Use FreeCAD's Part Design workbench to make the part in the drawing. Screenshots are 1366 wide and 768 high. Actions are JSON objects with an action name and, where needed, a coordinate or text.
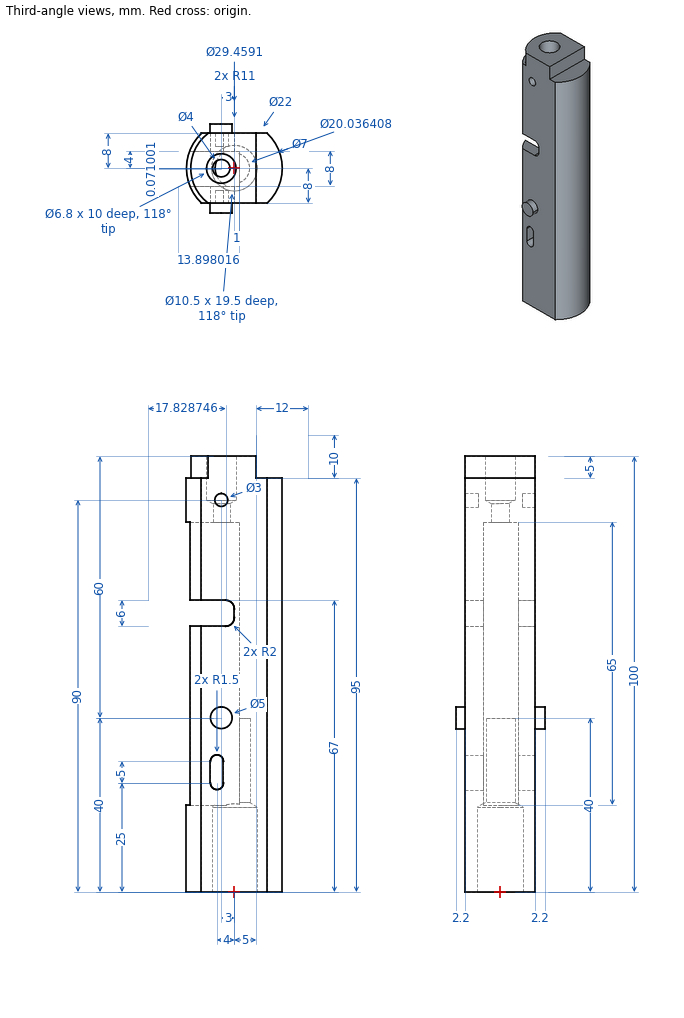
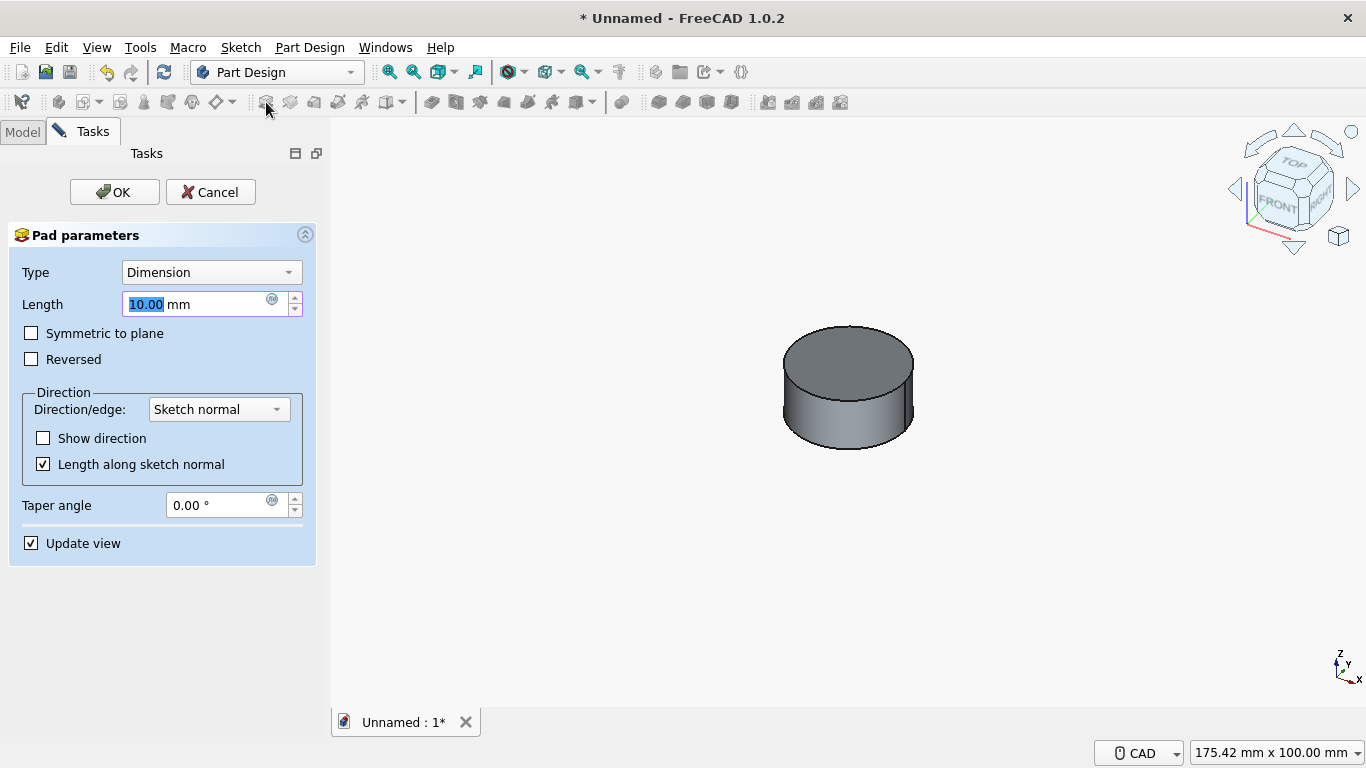
{"action": "type", "text": "100"}
{"action": "key", "text": "Tab"}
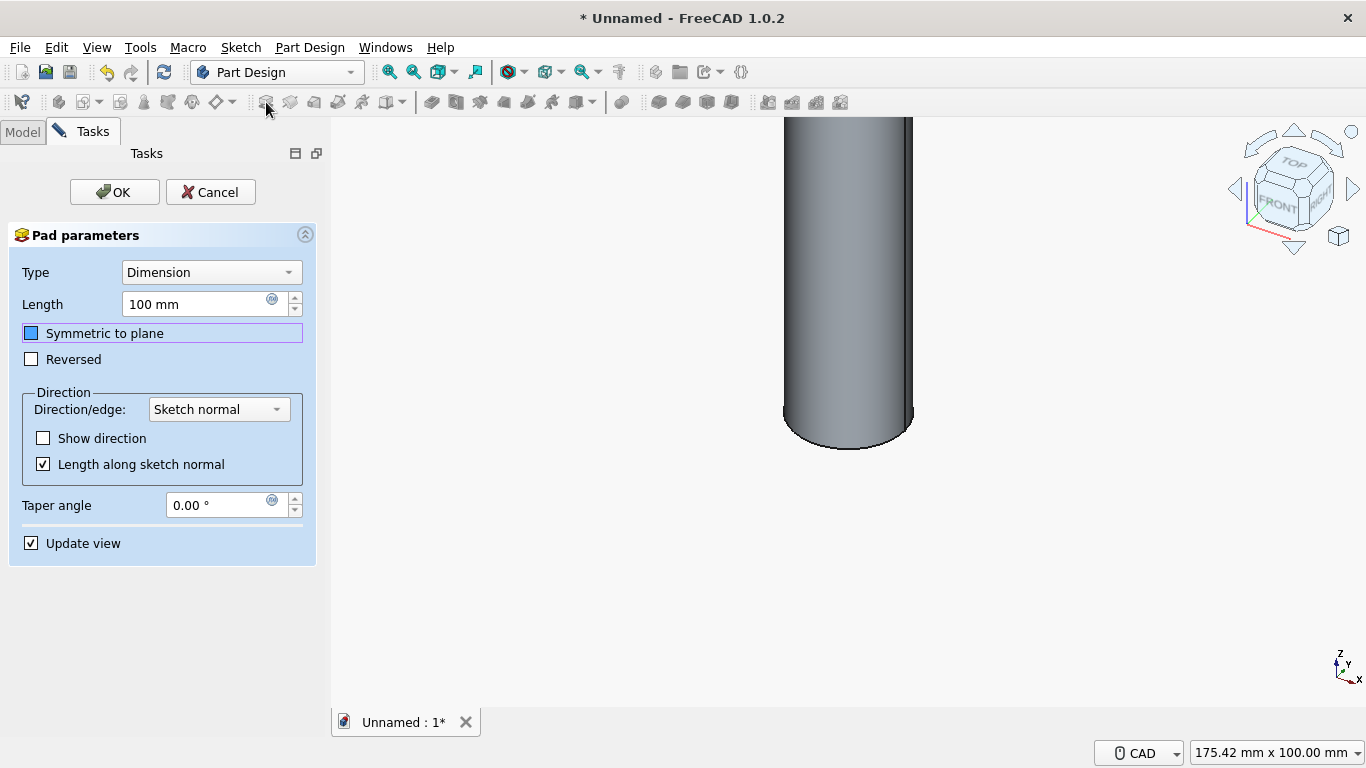
{"action": "left_click", "coordinate": [115, 192]}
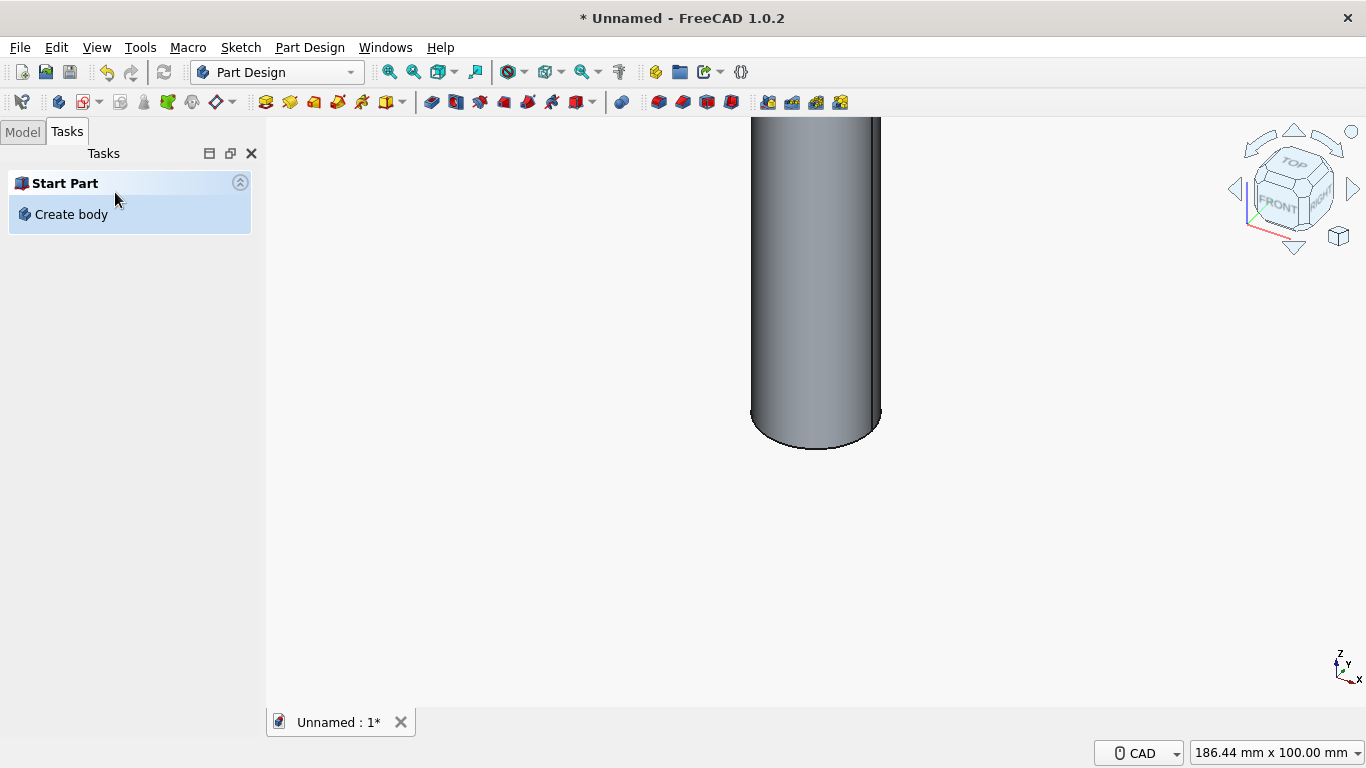
{"action": "key", "text": "v f"}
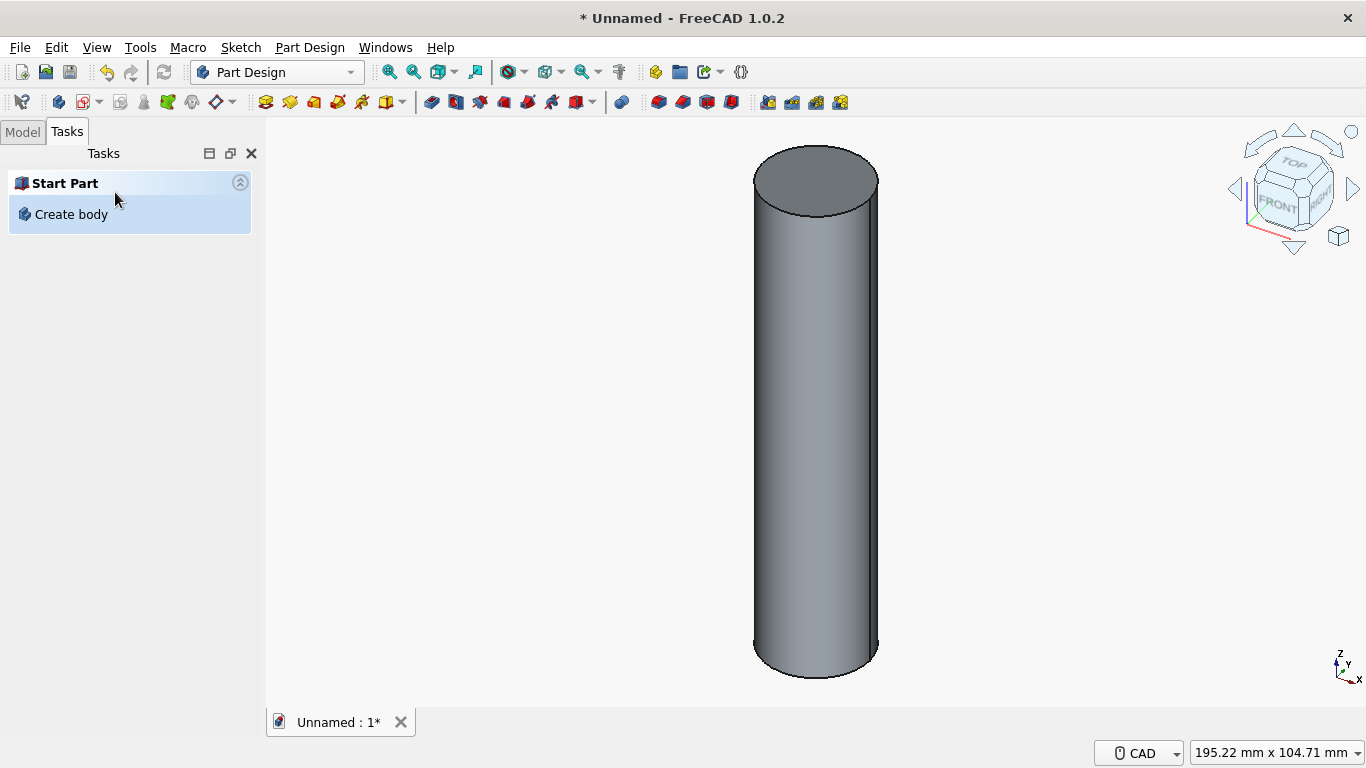
{"action": "left_click", "coordinate": [816, 180]}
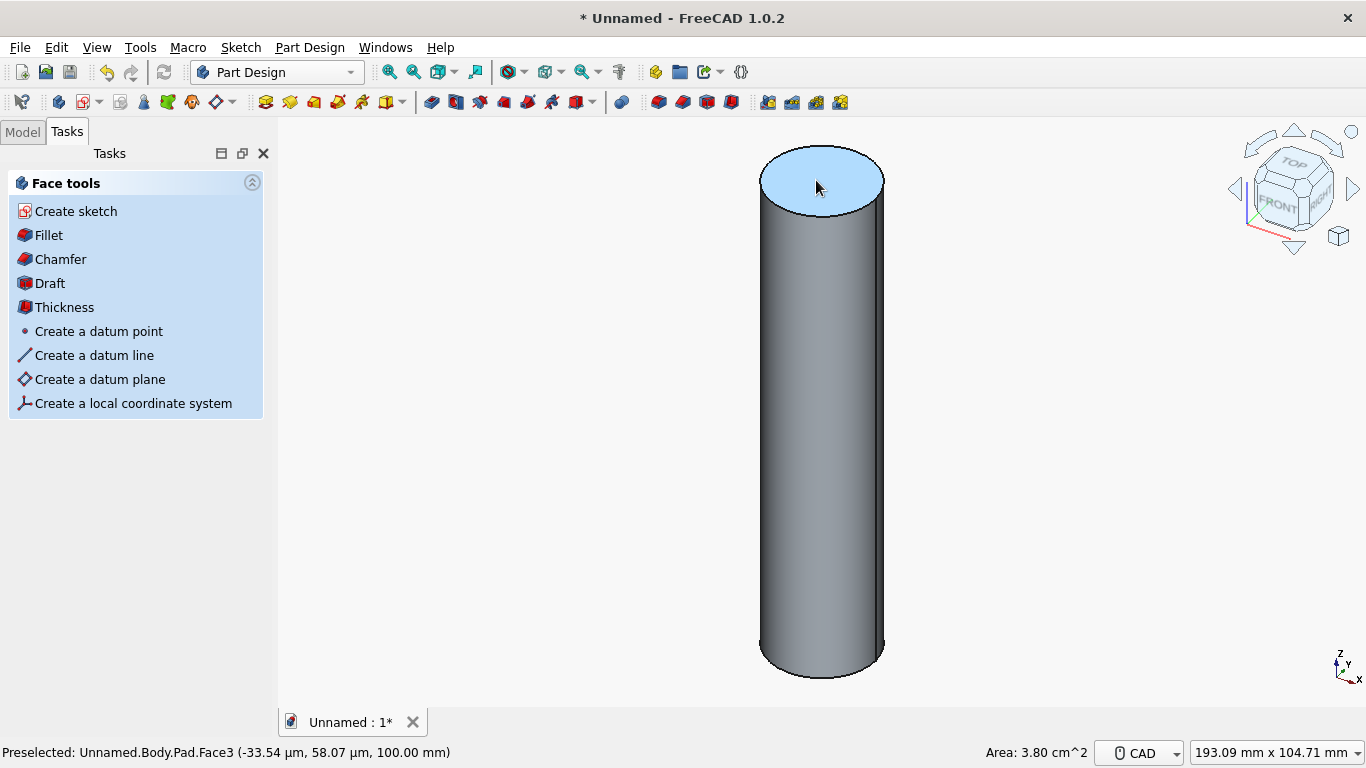
{"action": "left_click", "coordinate": [84, 102]}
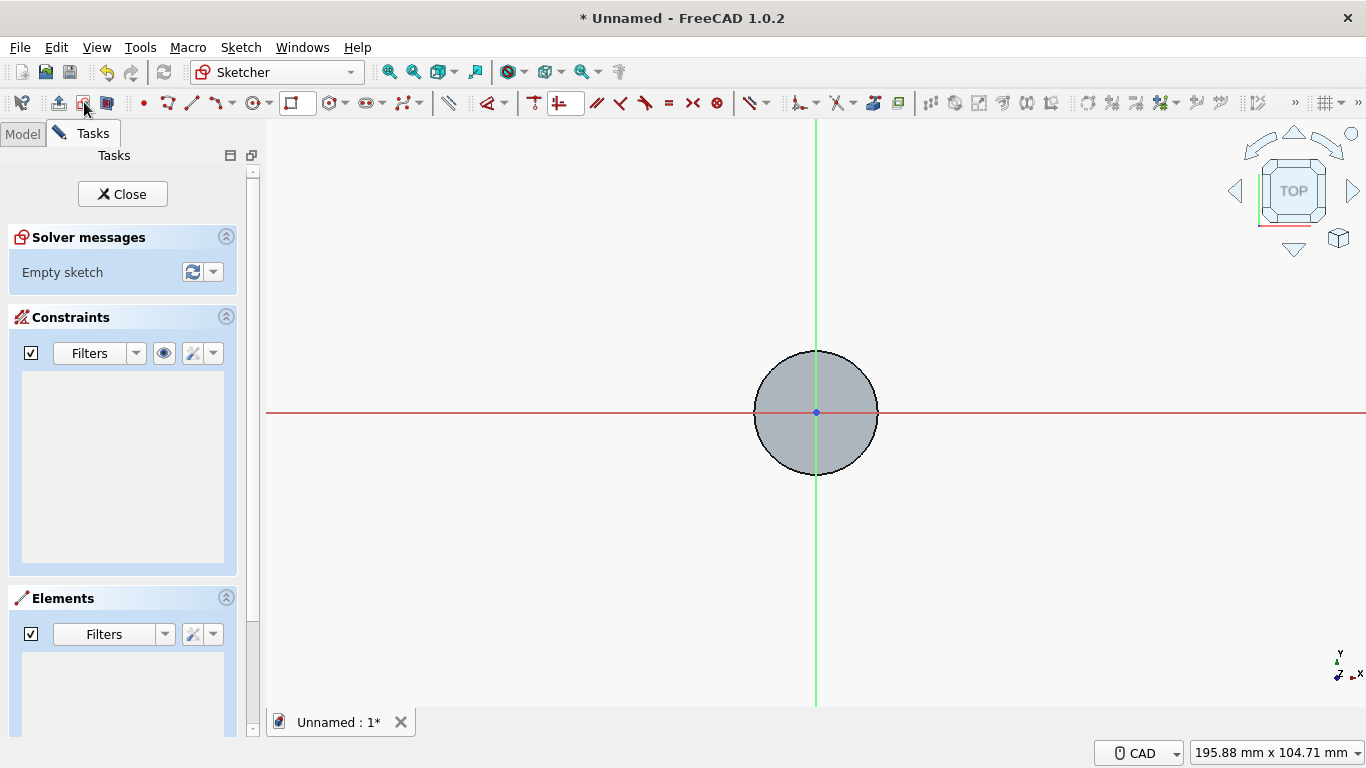
{"action": "scroll", "coordinate": [846, 413], "scroll_direction": "up", "scroll_amount": 6}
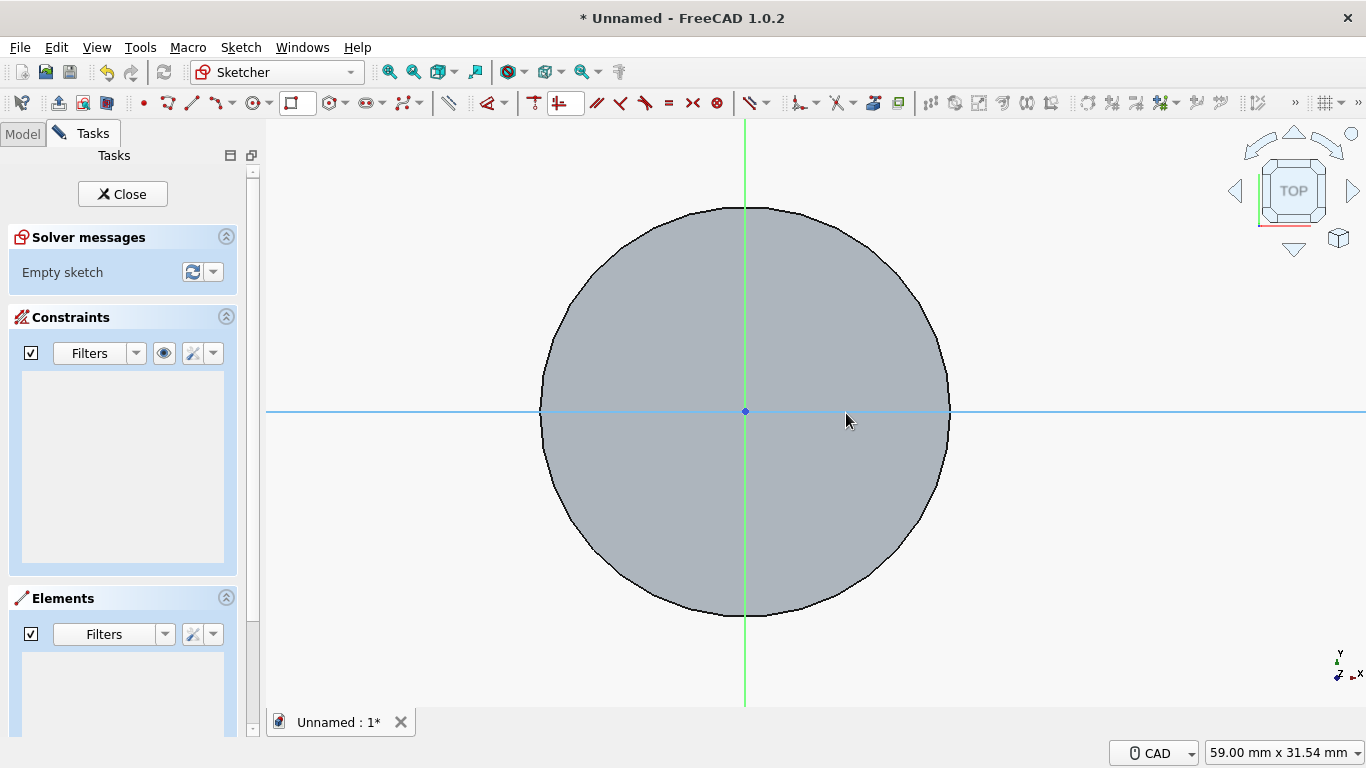
{"action": "key", "text": "g l"}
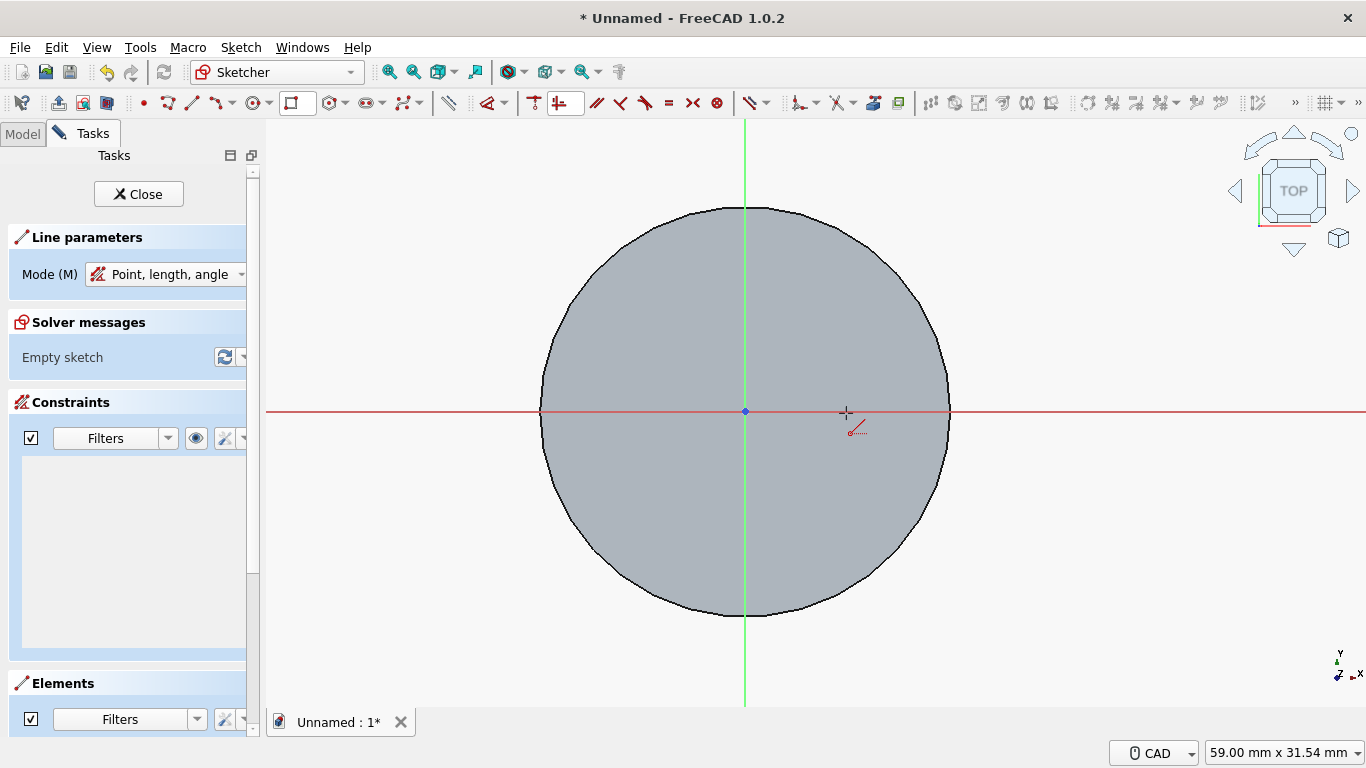
{"action": "left_click", "coordinate": [604, 263]}
{"action": "left_click", "coordinate": [886, 263]}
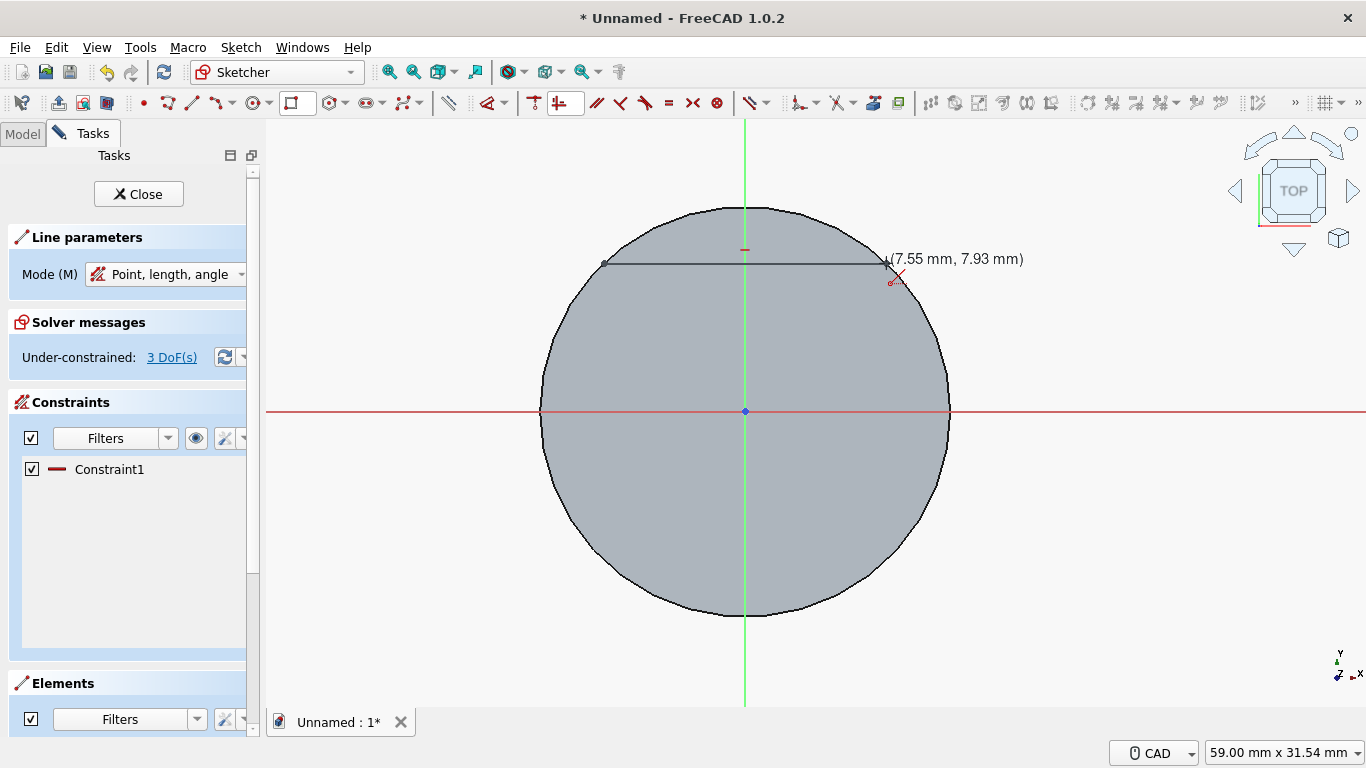
{"action": "left_click", "coordinate": [216, 104]}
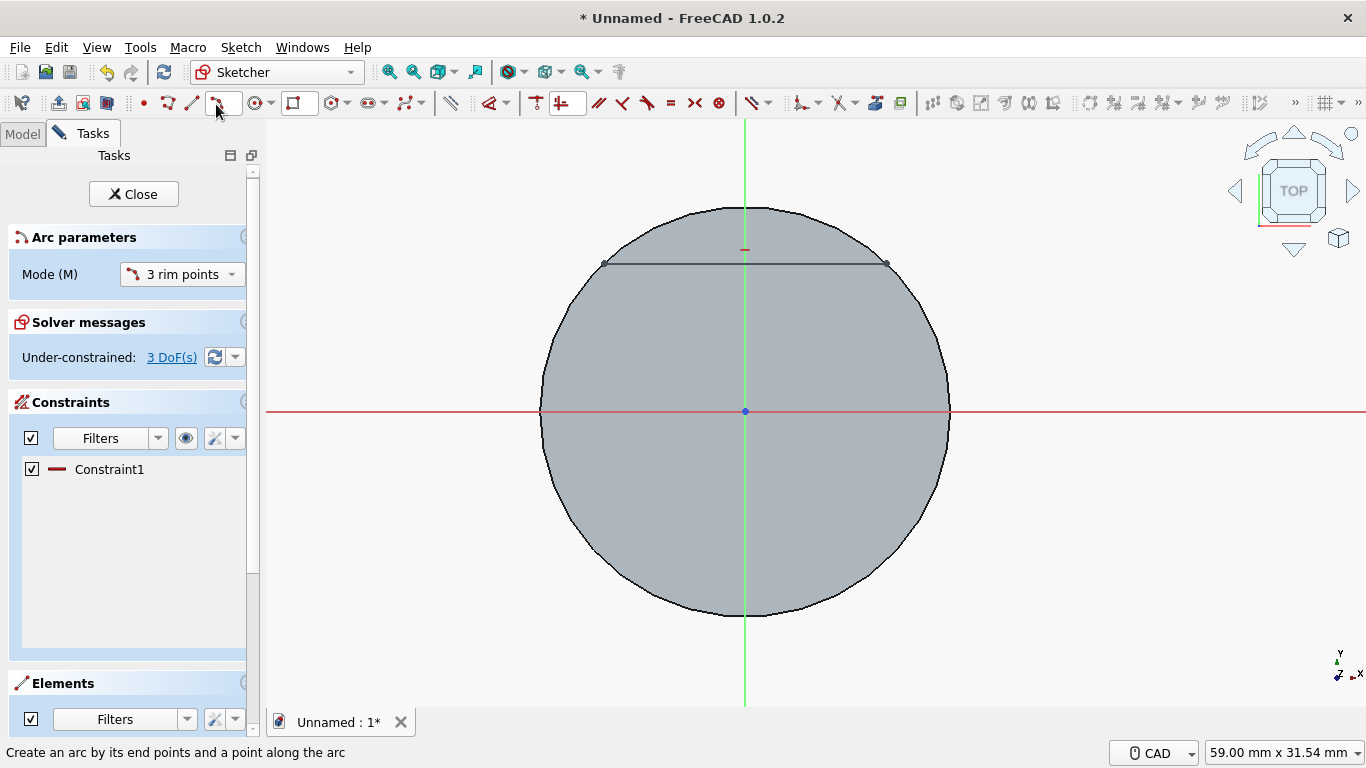
{"action": "left_click", "coordinate": [886, 264]}
{"action": "left_click", "coordinate": [604, 264]}
{"action": "left_click", "coordinate": [776, 209]}